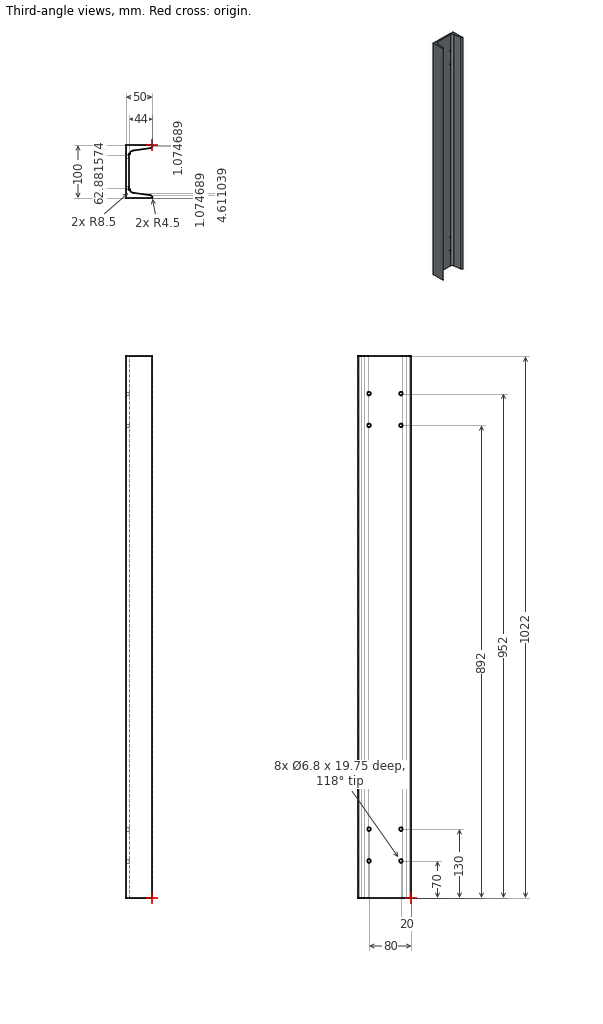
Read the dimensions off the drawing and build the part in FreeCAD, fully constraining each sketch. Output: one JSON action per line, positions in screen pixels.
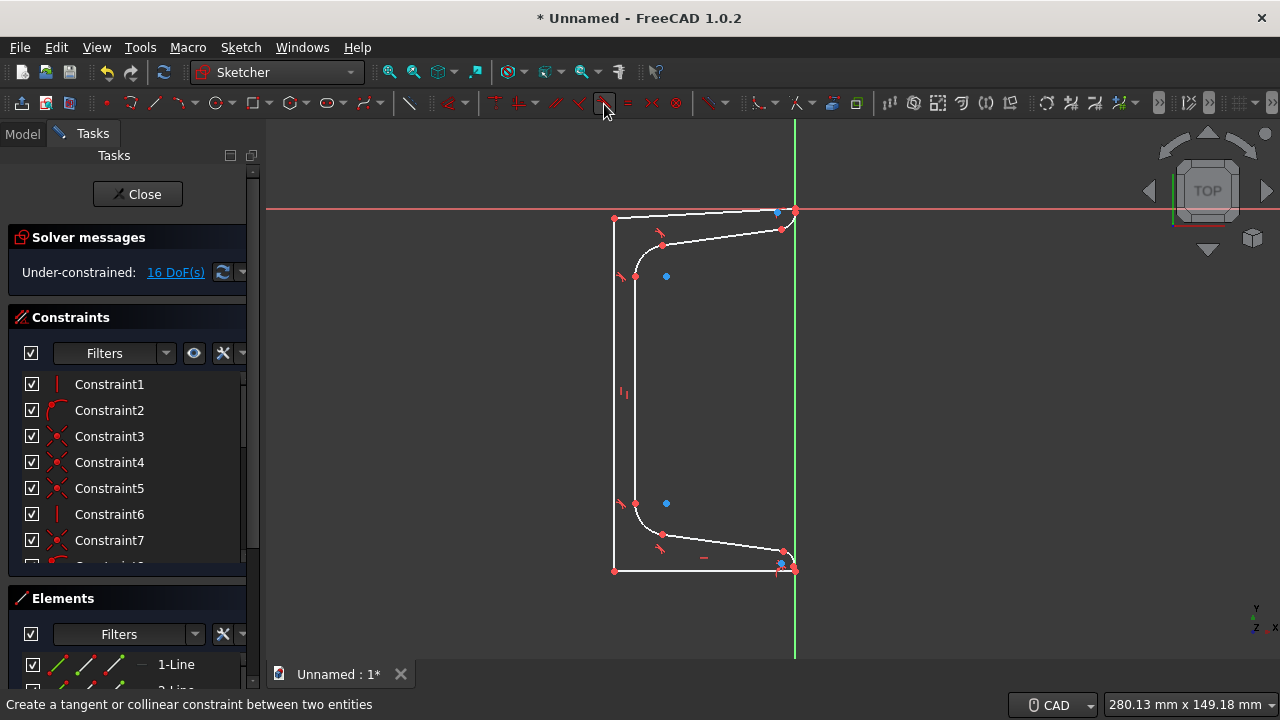
{"action": "left_click", "coordinate": [698, 241]}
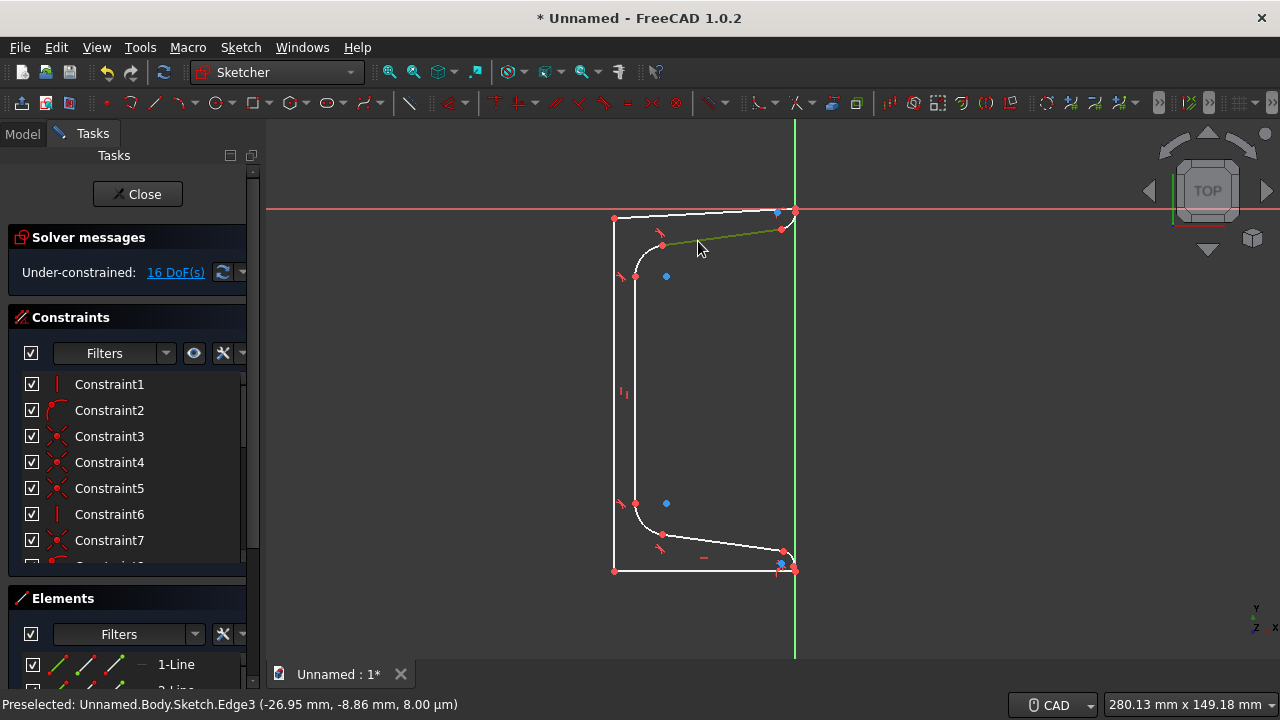
{"action": "scroll", "coordinate": [794, 220], "scroll_direction": "up", "scroll_amount": 4}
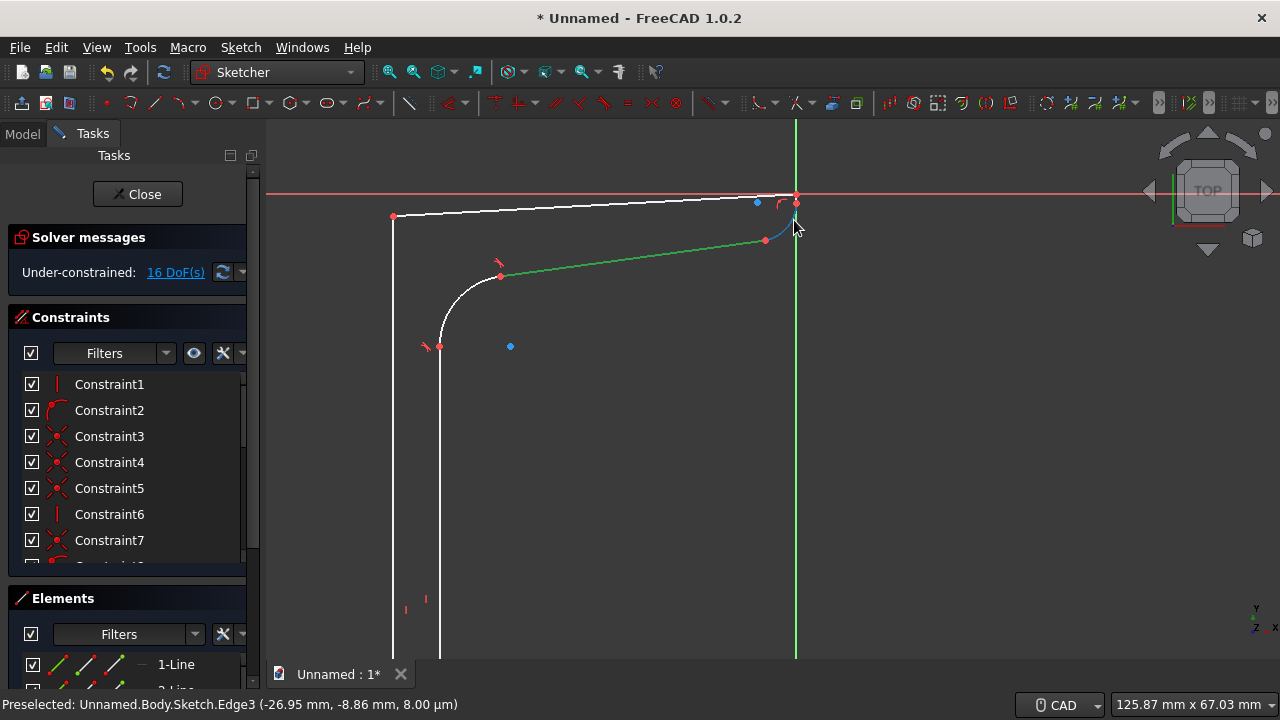
{"action": "left_click", "coordinate": [793, 219]}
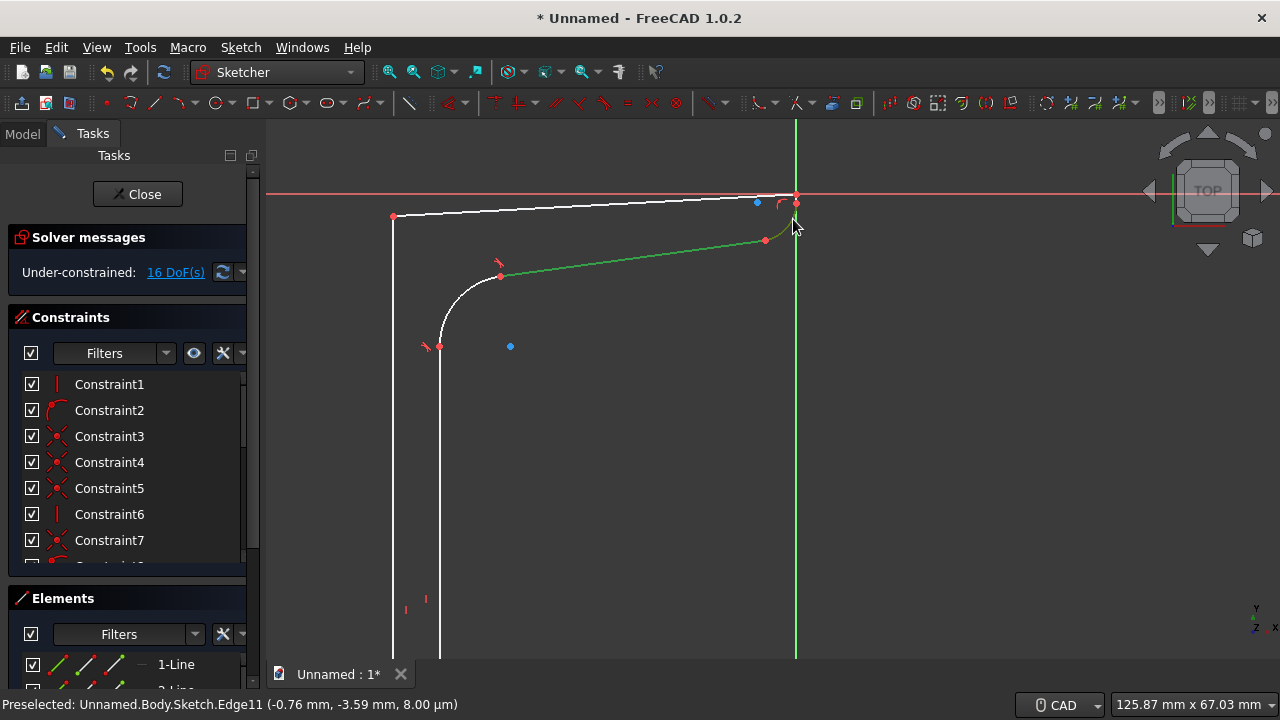
{"action": "left_click", "coordinate": [604, 104]}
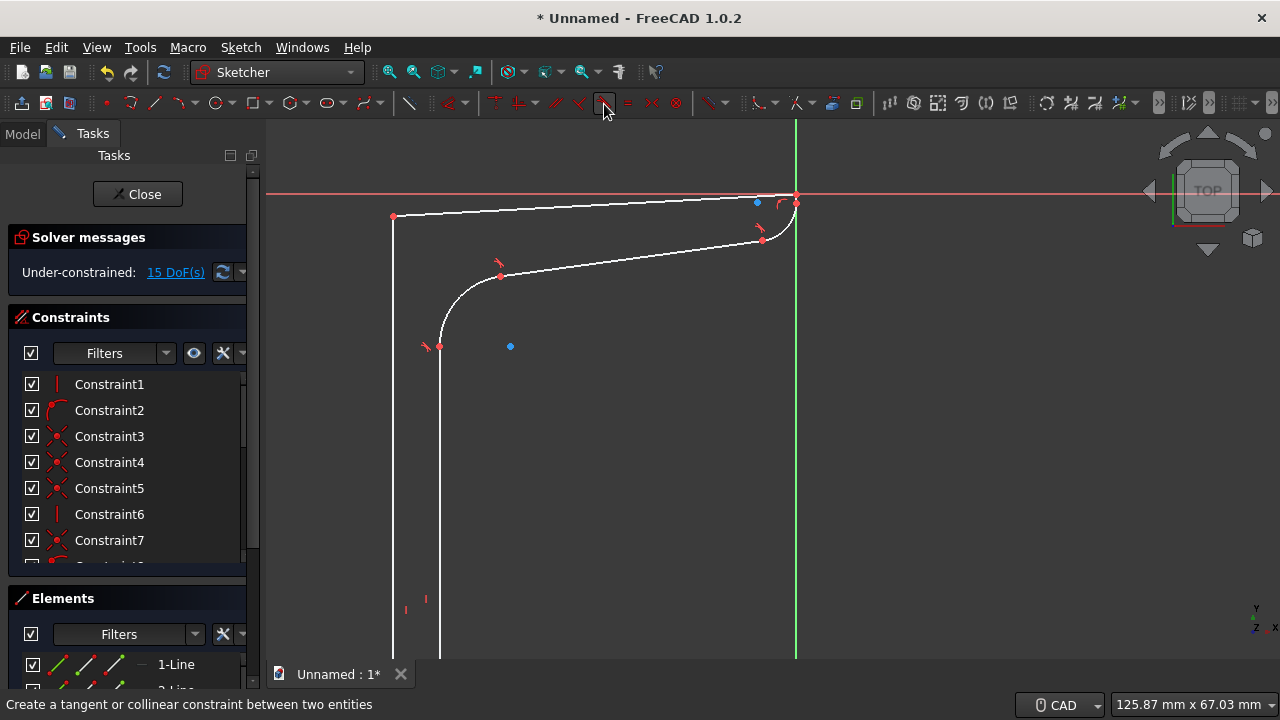
{"action": "scroll", "coordinate": [796, 199], "scroll_direction": "up", "scroll_amount": 6}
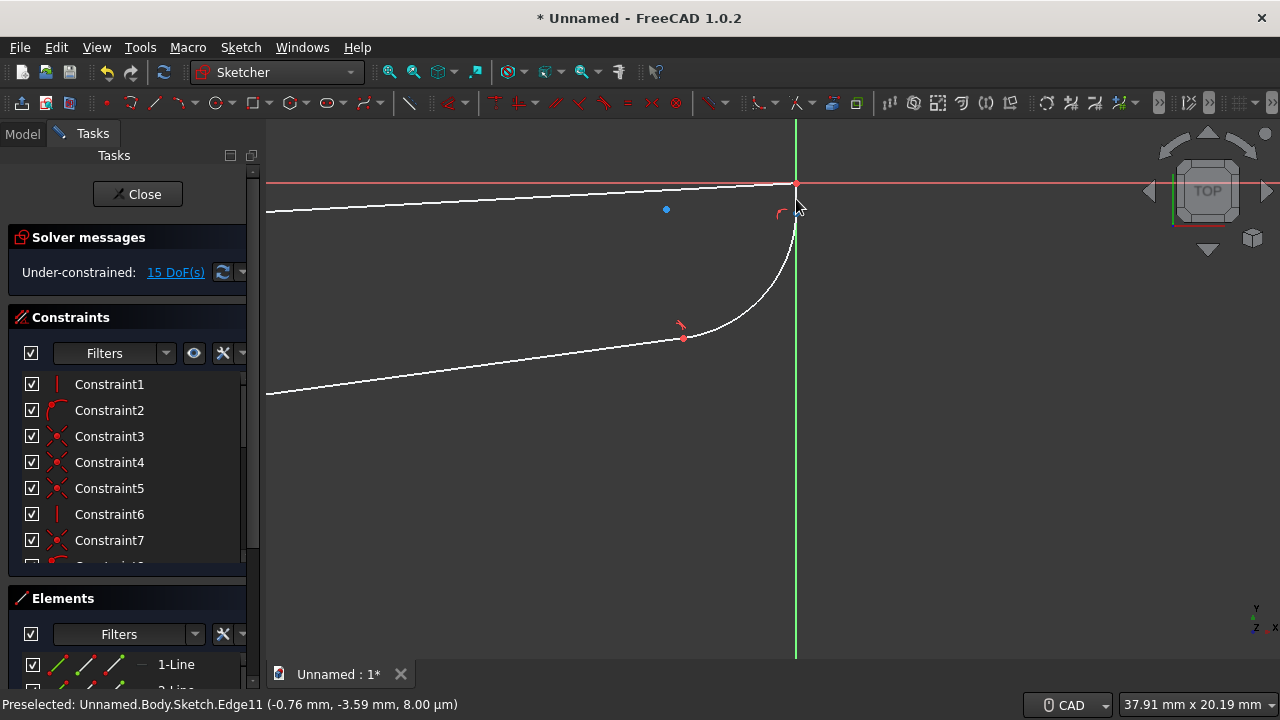
{"action": "left_click", "coordinate": [796, 199]}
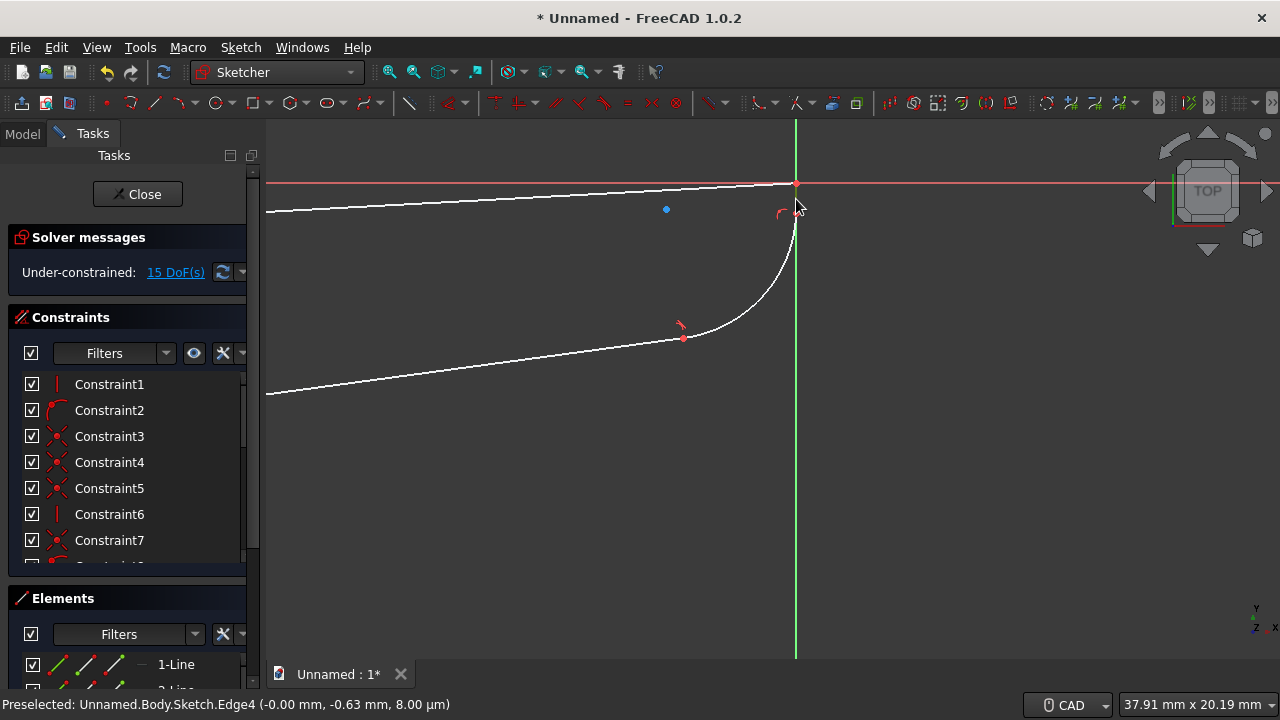
{"action": "scroll", "coordinate": [795, 212], "scroll_direction": "down", "scroll_amount": 10}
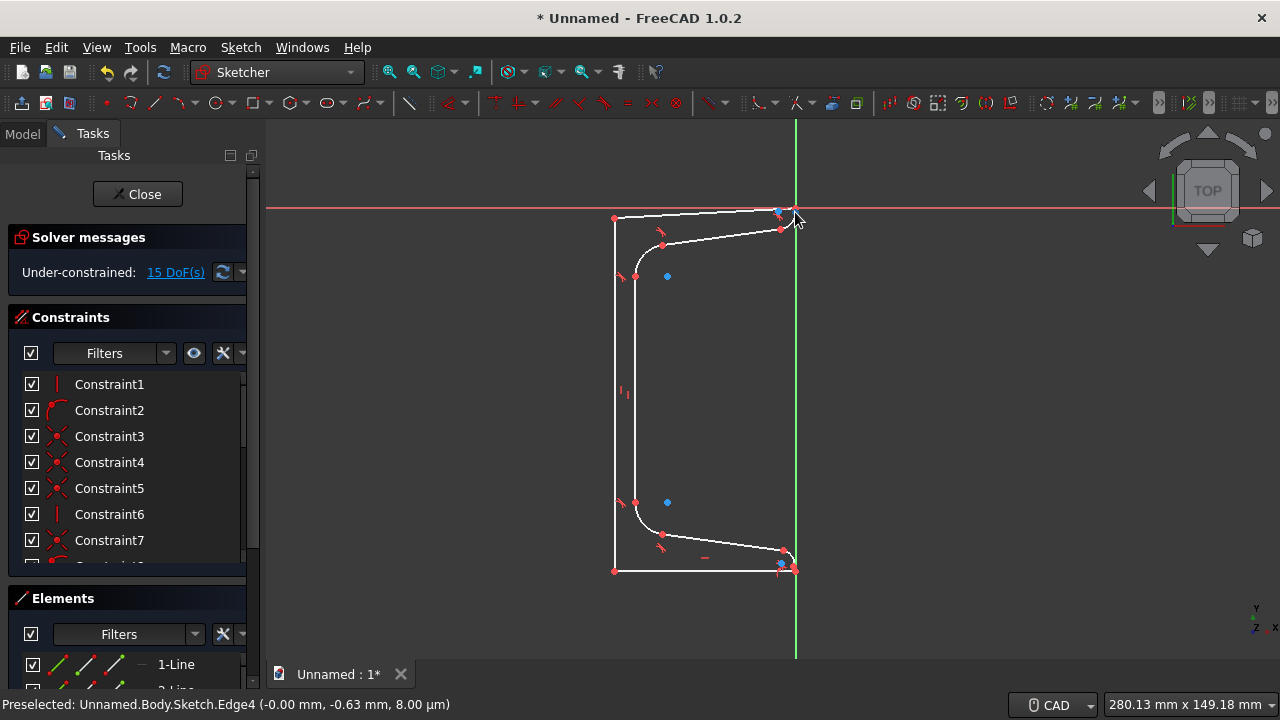
{"action": "scroll", "coordinate": [787, 227], "scroll_direction": "up", "scroll_amount": 4}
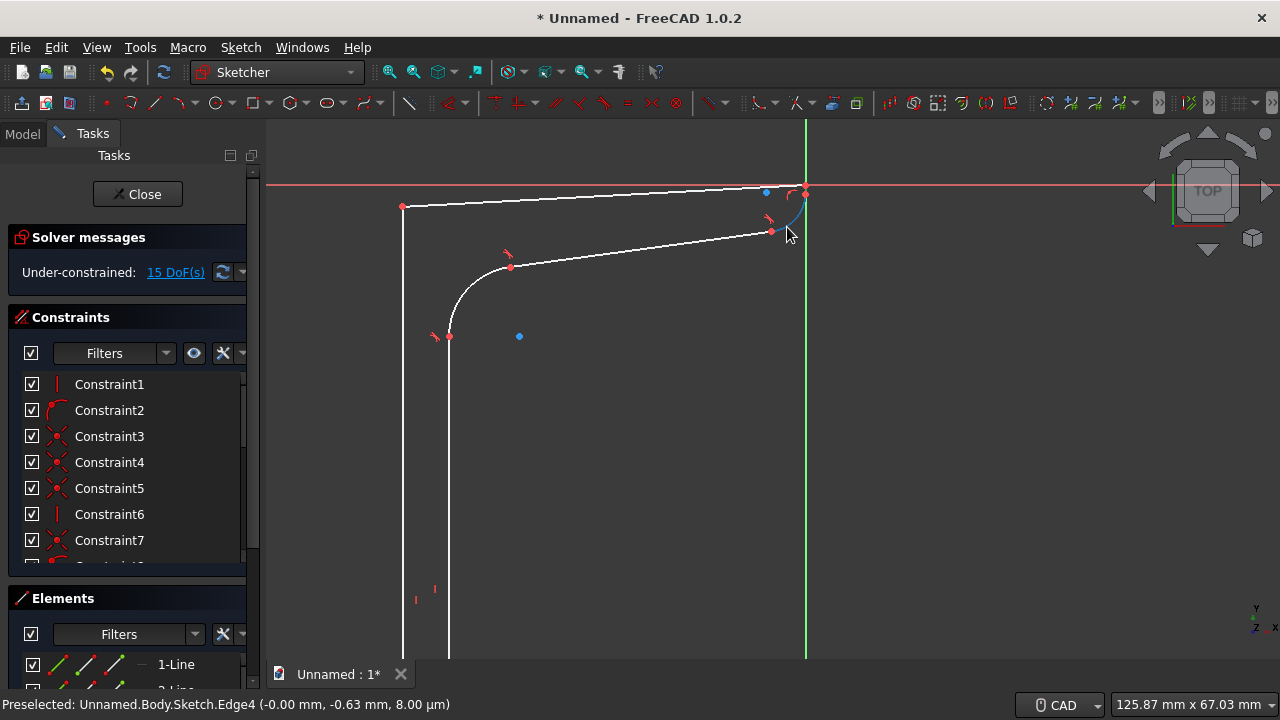
{"action": "left_click", "coordinate": [787, 226]}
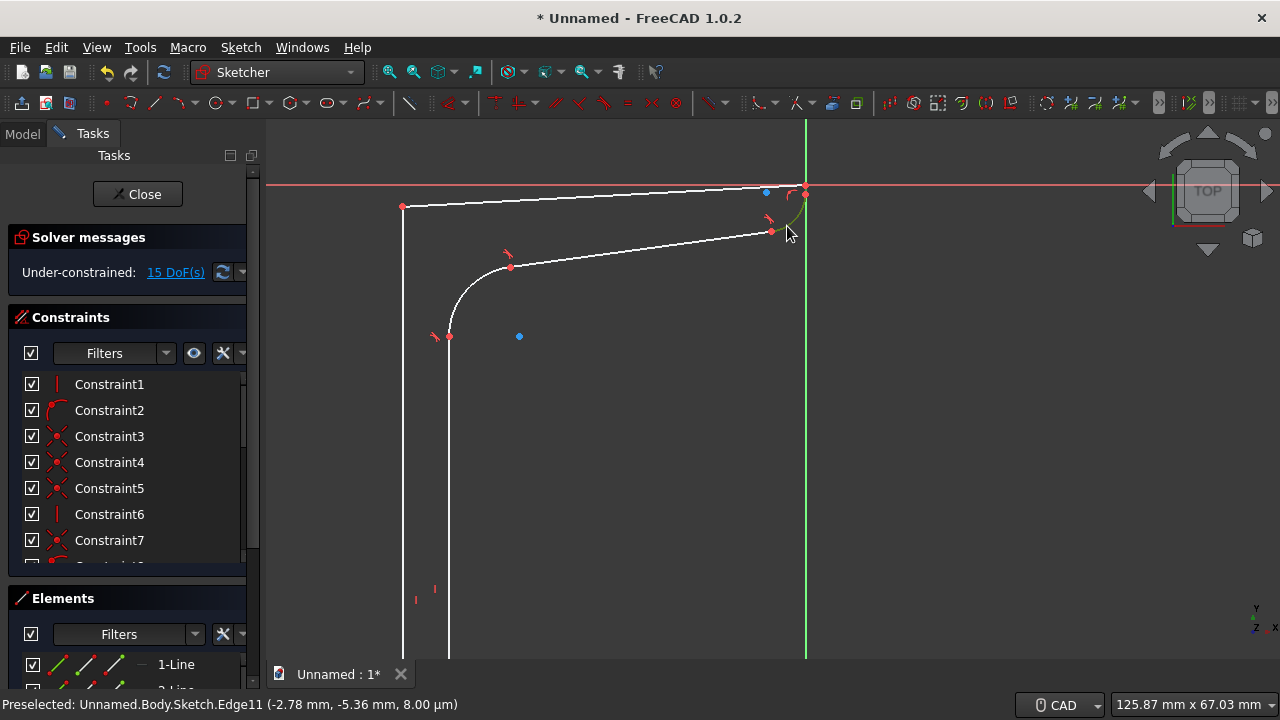
{"action": "left_click", "coordinate": [604, 104]}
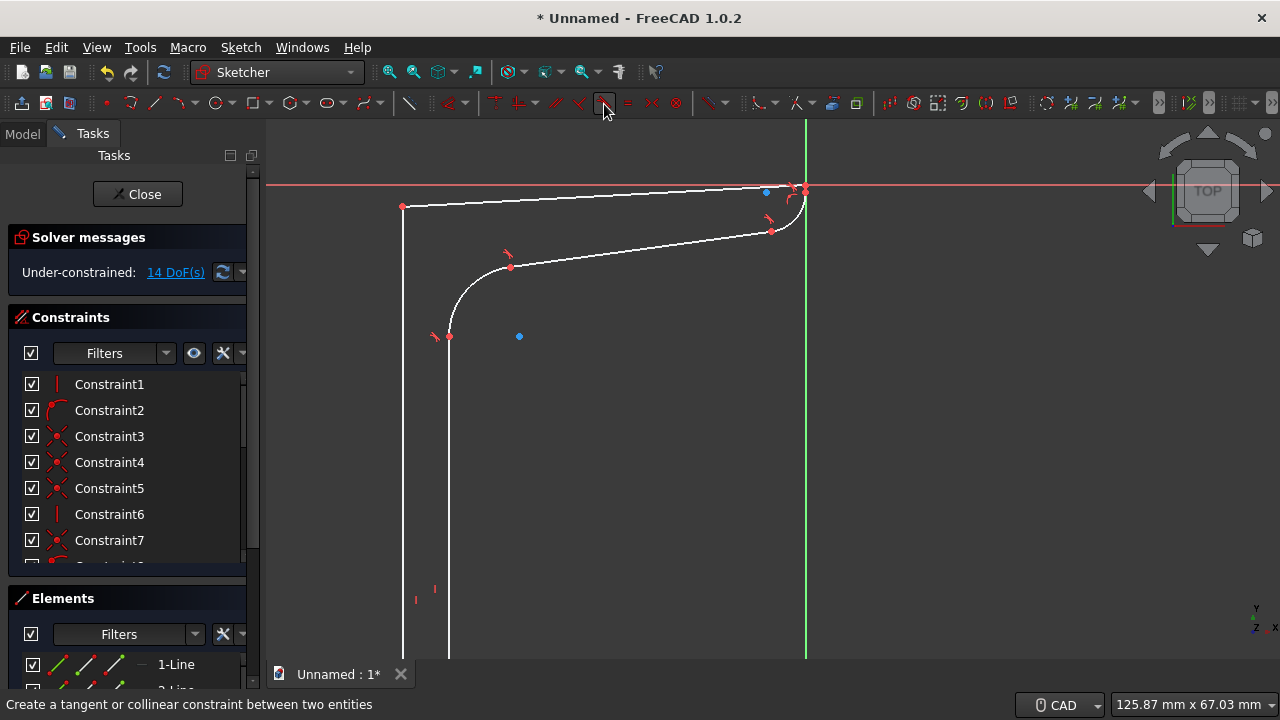
{"action": "scroll", "coordinate": [786, 227], "scroll_direction": "down", "scroll_amount": 4}